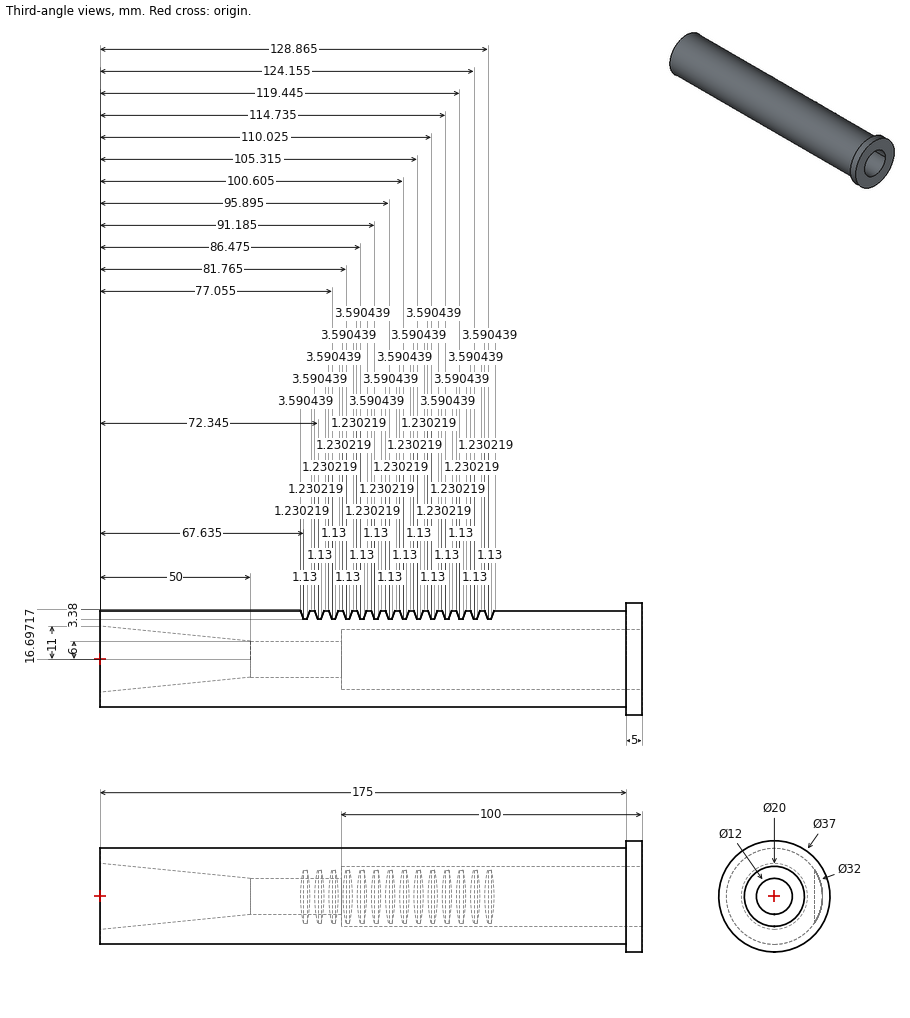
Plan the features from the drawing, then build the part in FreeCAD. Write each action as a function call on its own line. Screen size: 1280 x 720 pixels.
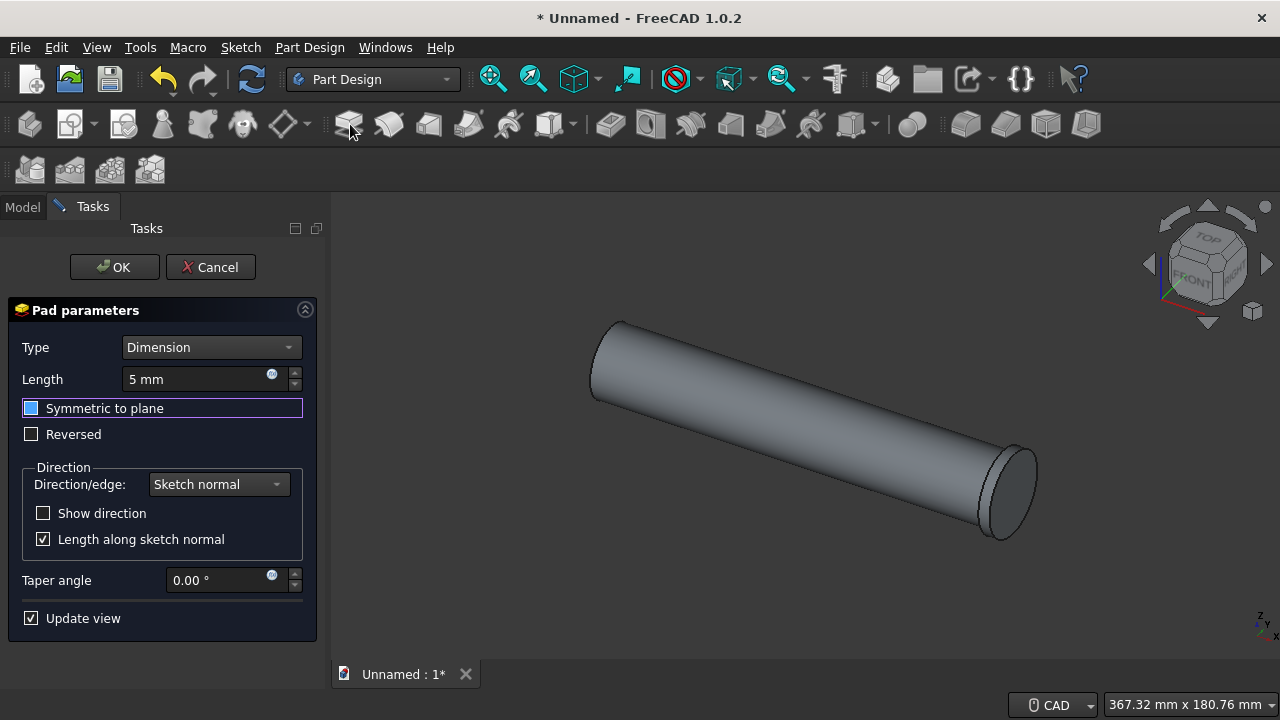
click(115, 267)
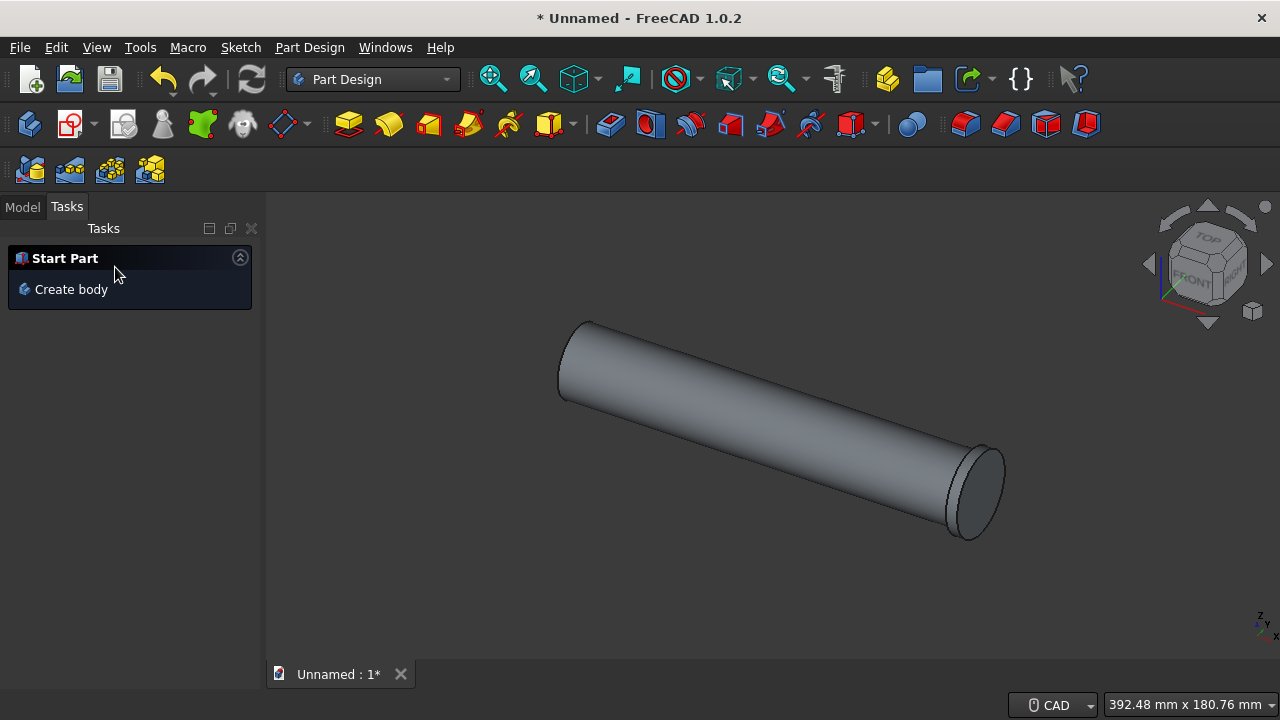
click(981, 493)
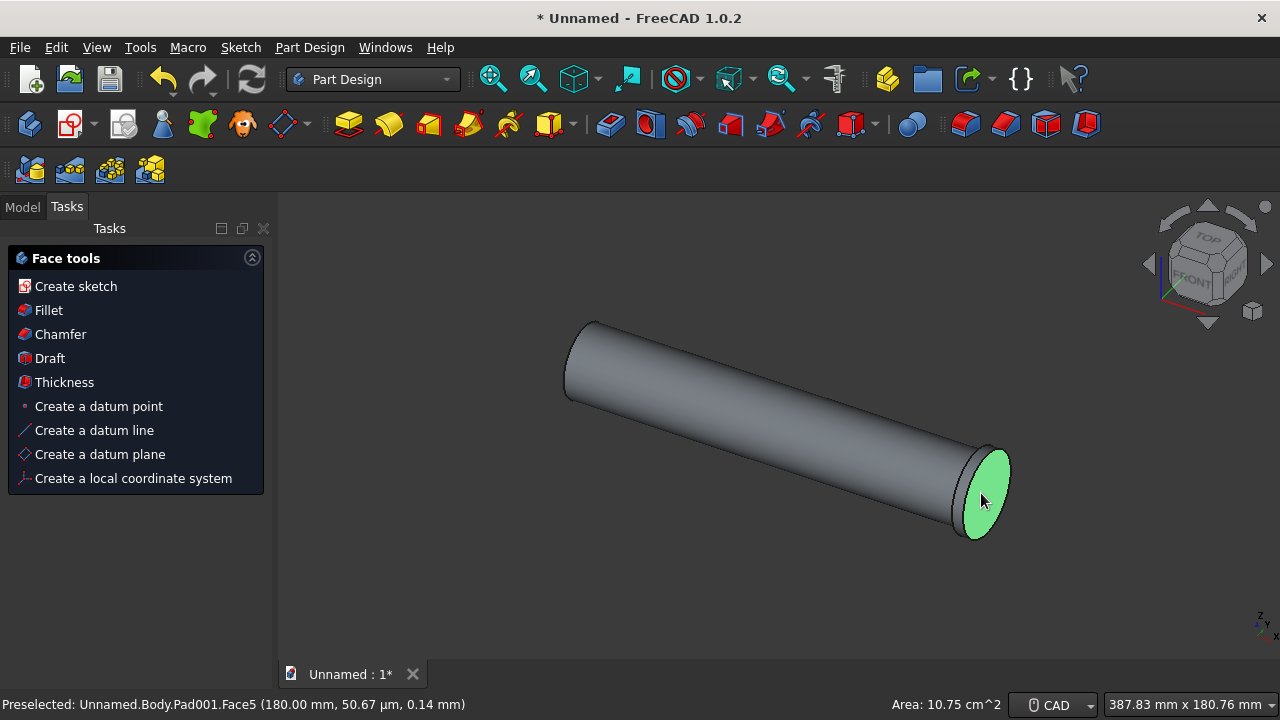
click(70, 124)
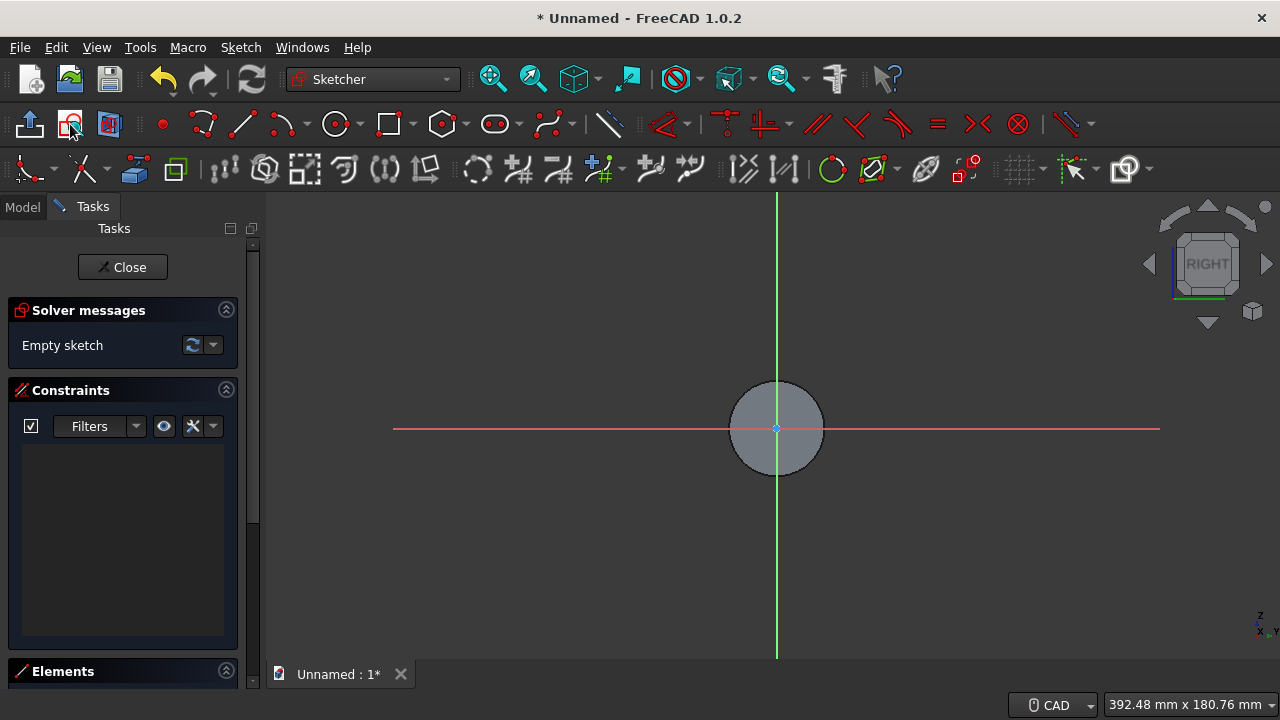
scroll(791, 429, up, 9)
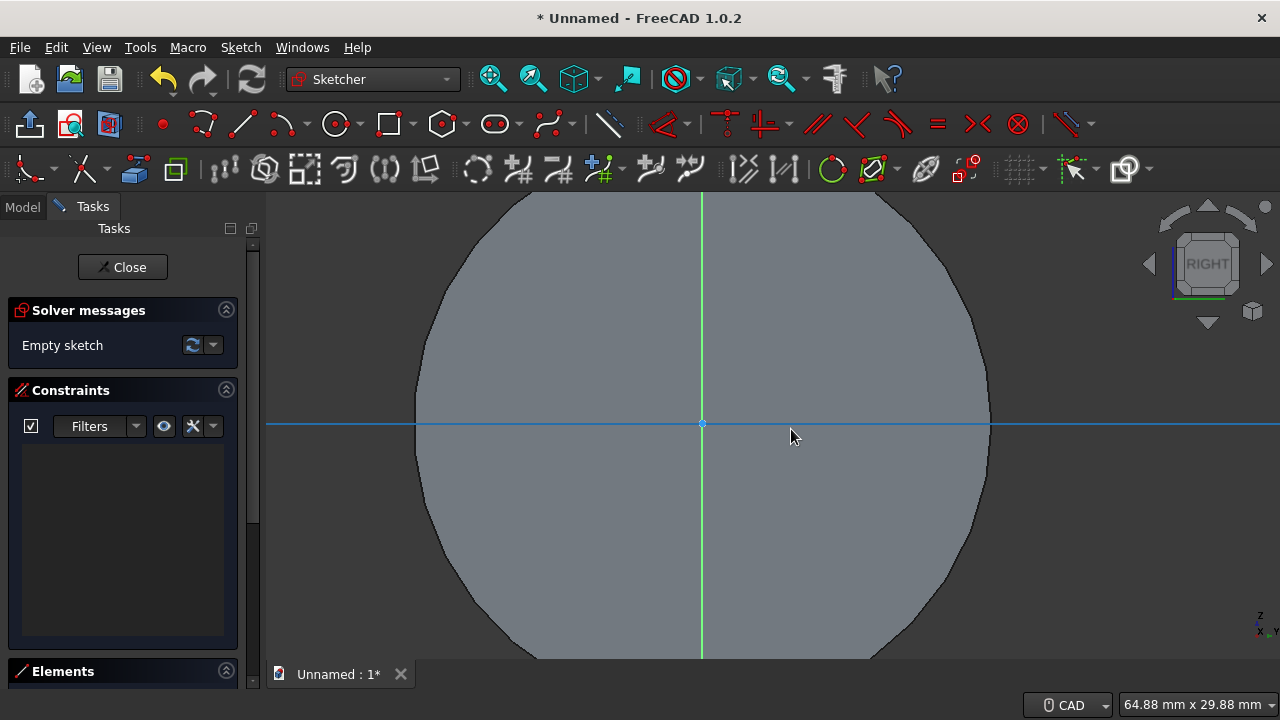
click(336, 124)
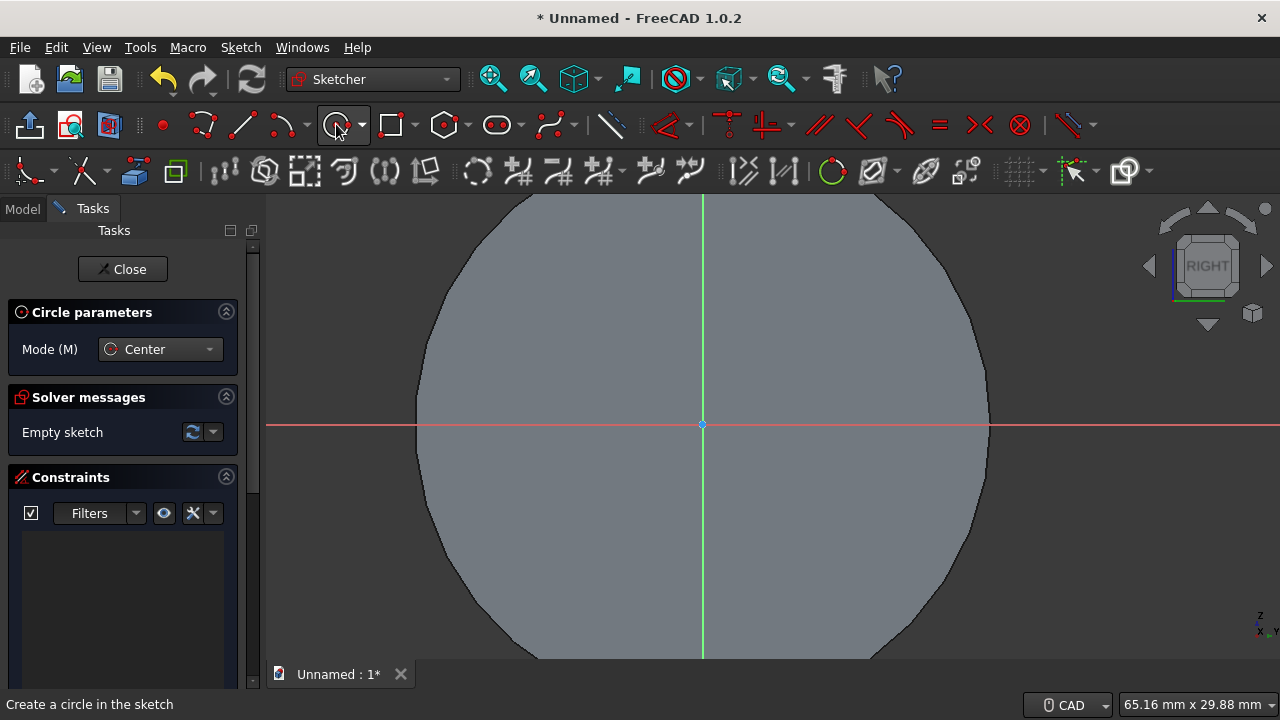
click(703, 425)
move(813, 315)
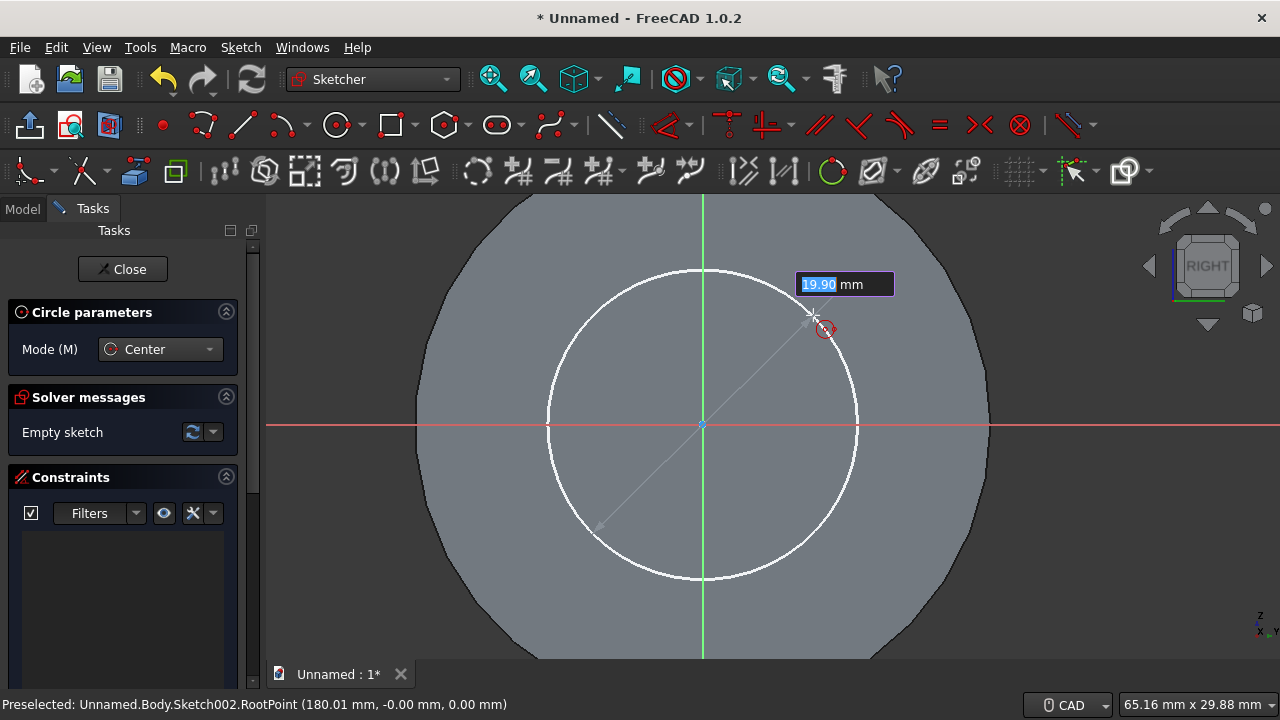
text(20)
key(Return)
key(Escape)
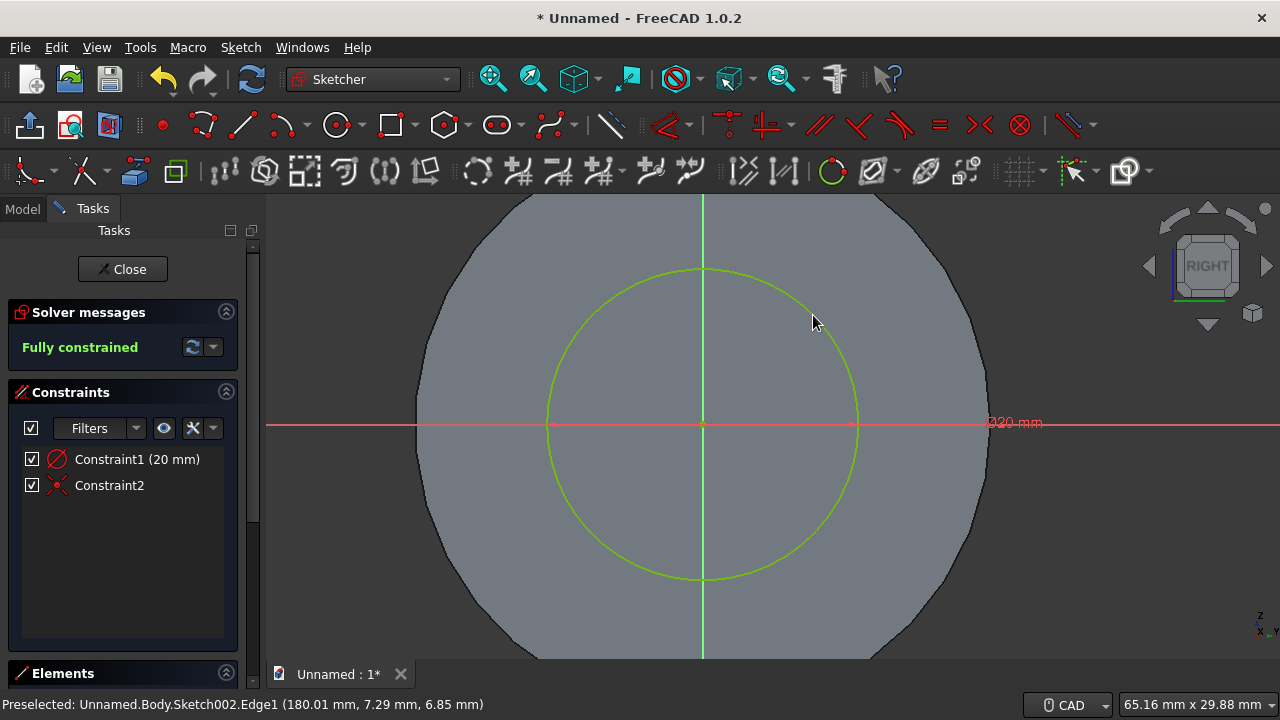
click(123, 269)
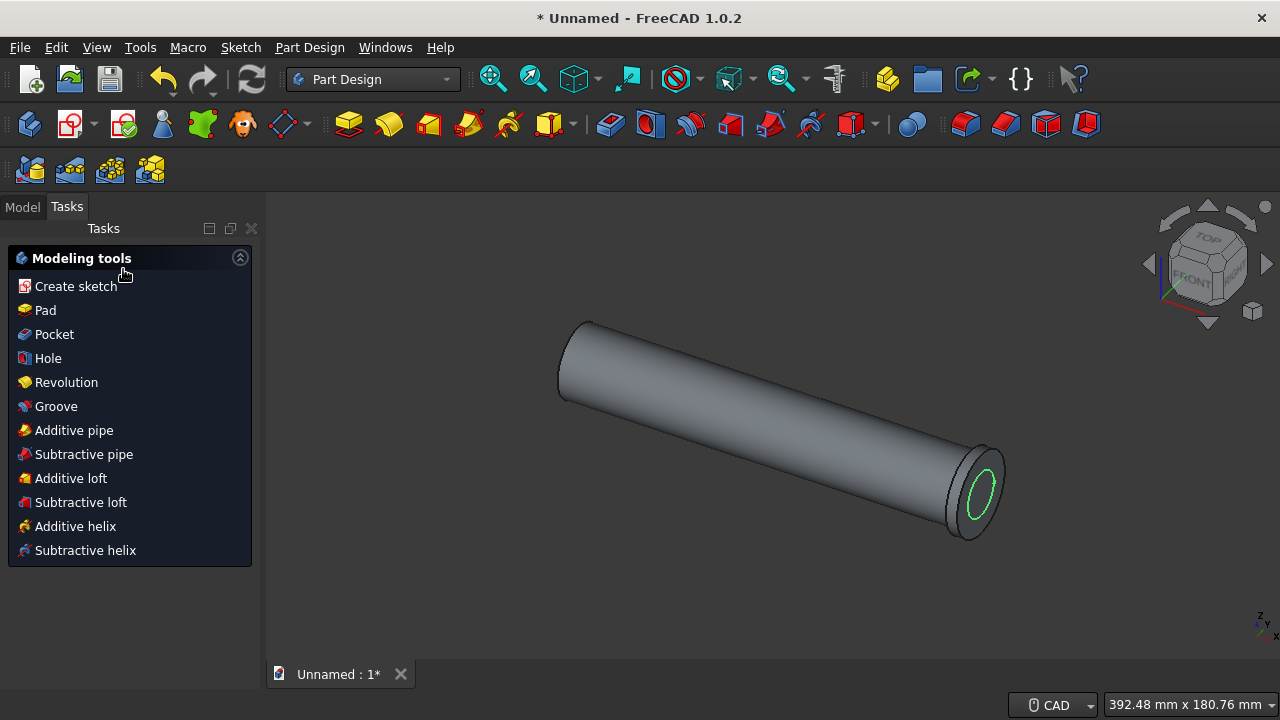
click(612, 124)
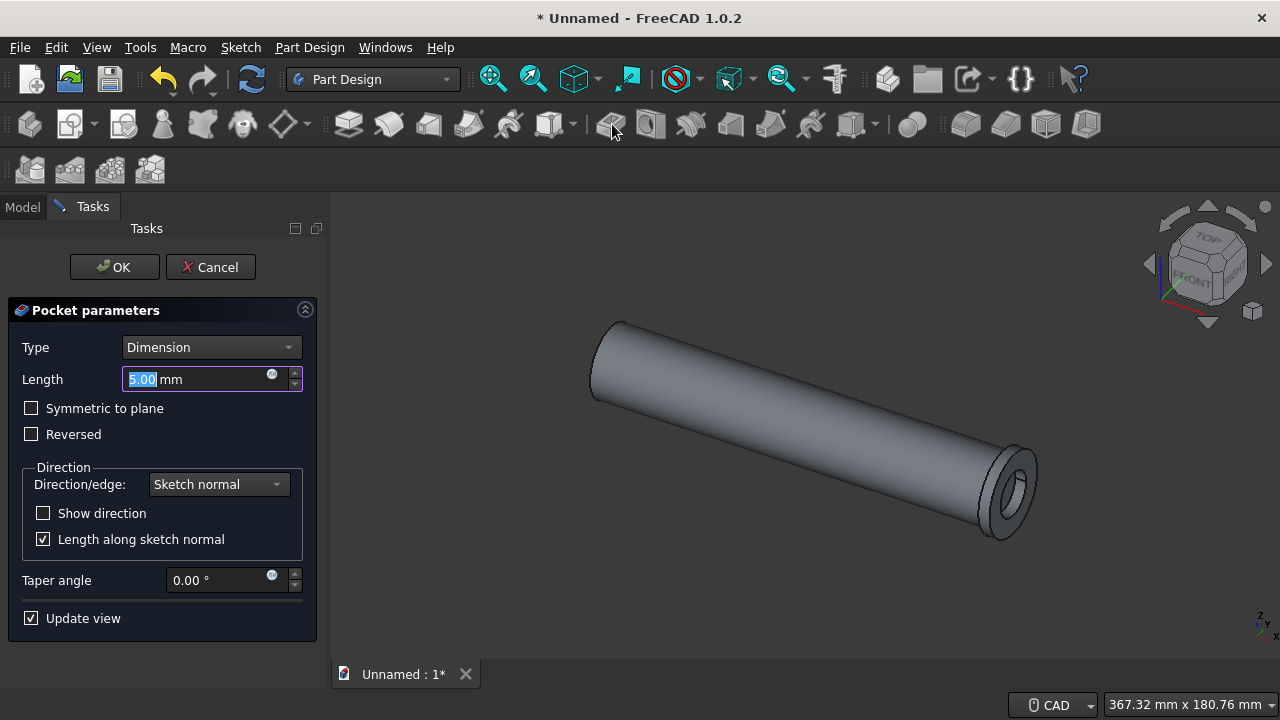
text(100)
key(Tab)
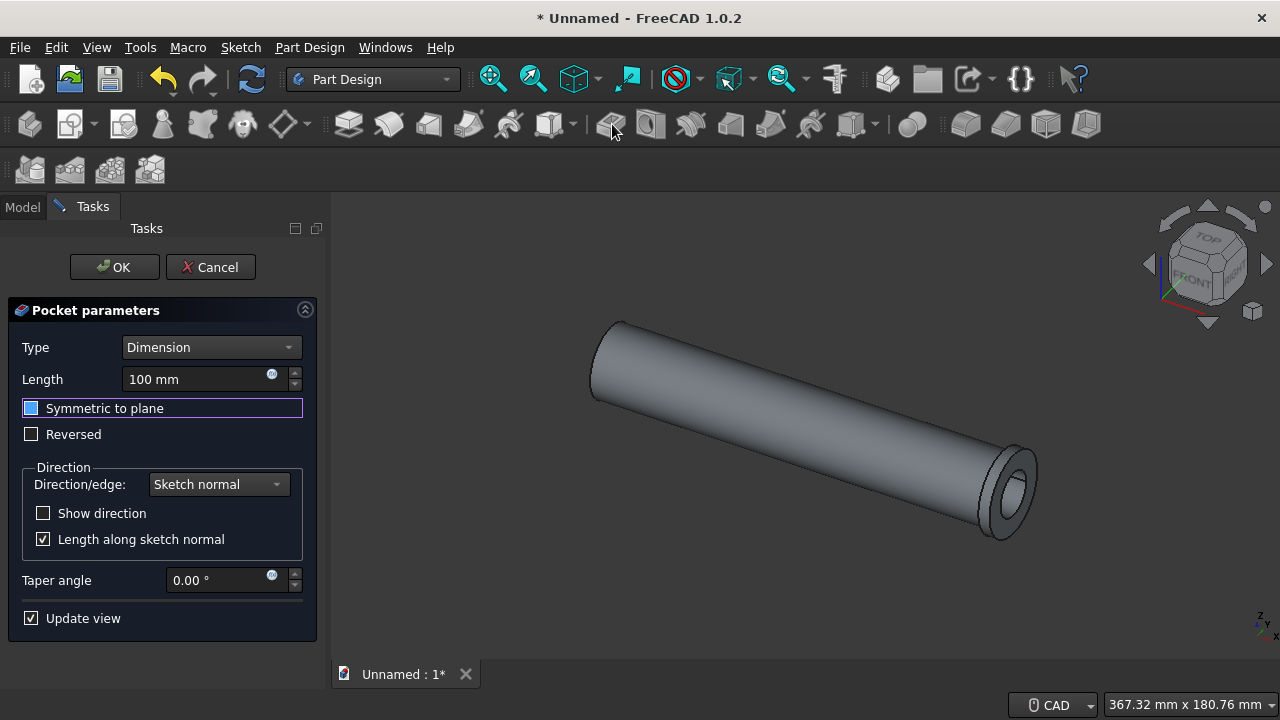
click(115, 267)